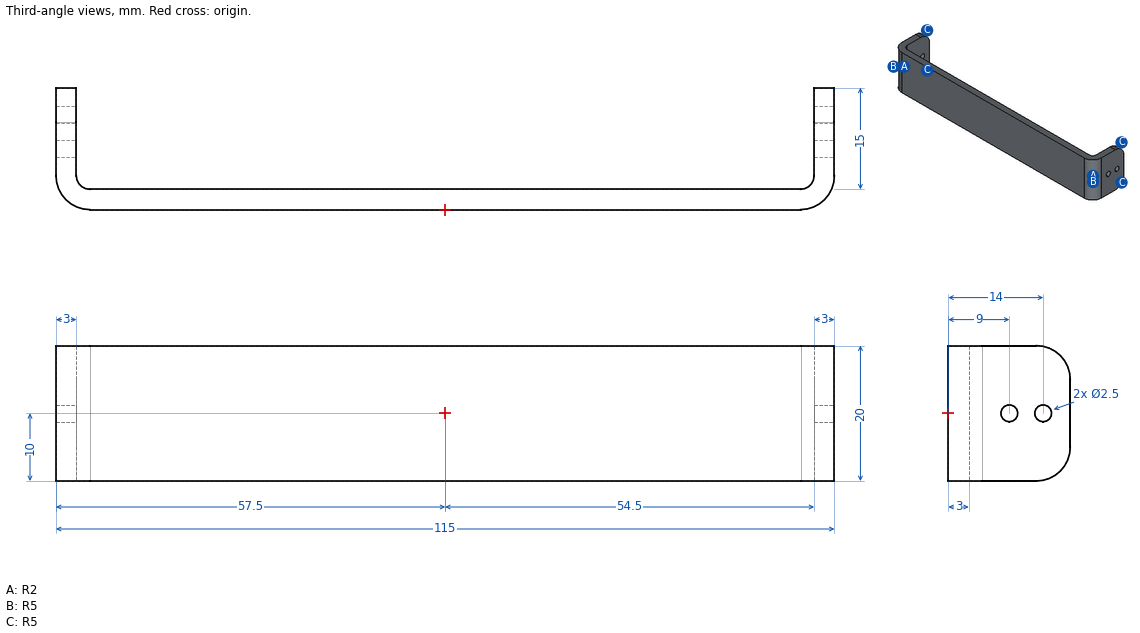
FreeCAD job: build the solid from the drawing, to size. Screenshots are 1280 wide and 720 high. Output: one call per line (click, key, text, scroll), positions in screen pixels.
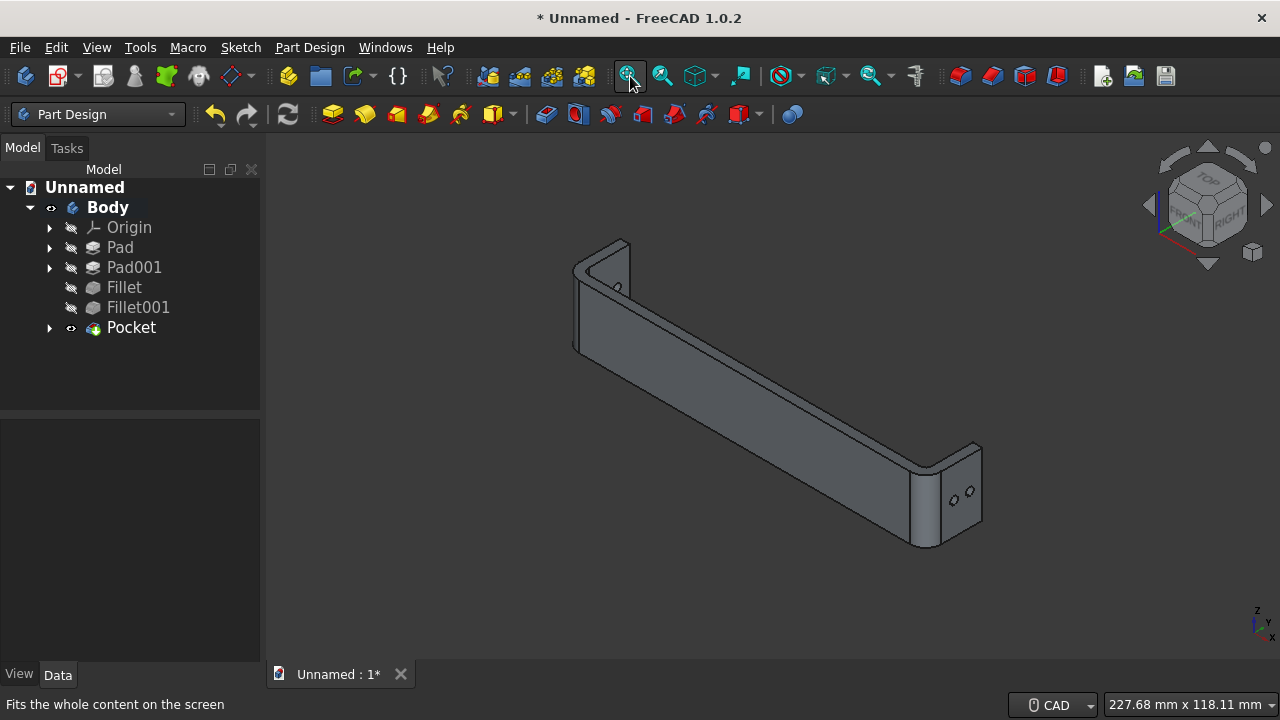
scroll(625, 240, up, 6)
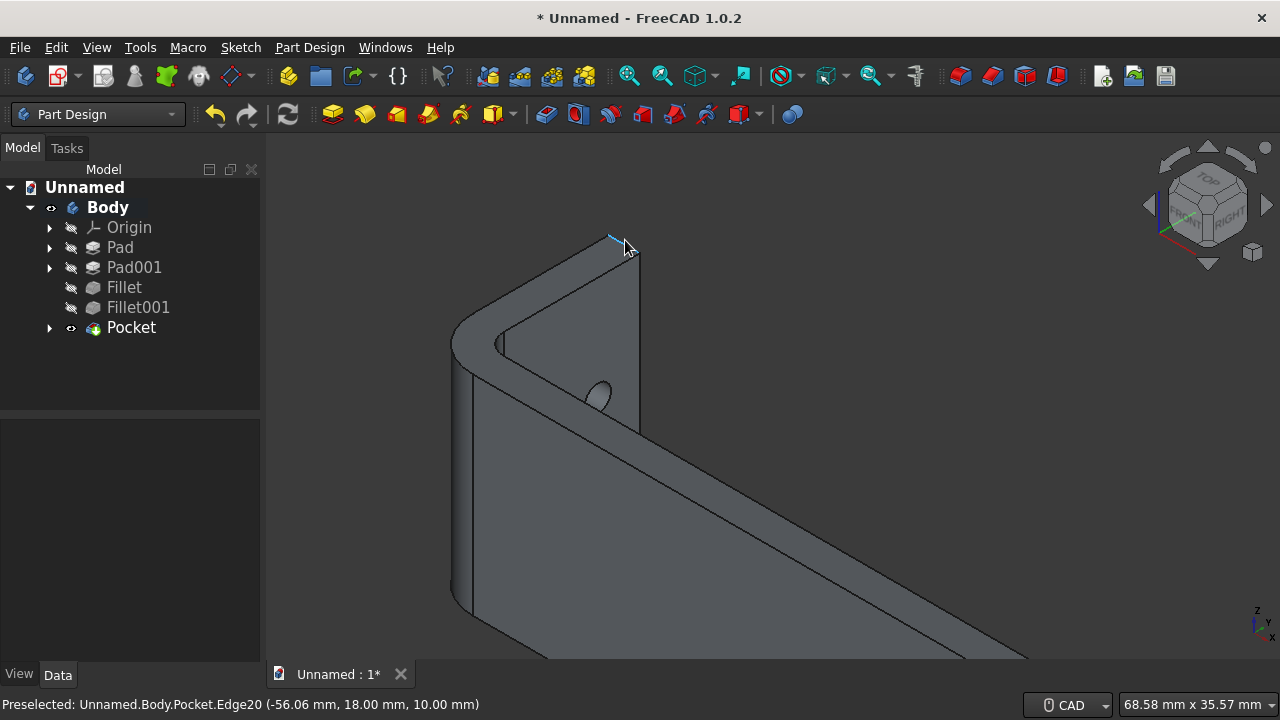
click(630, 76)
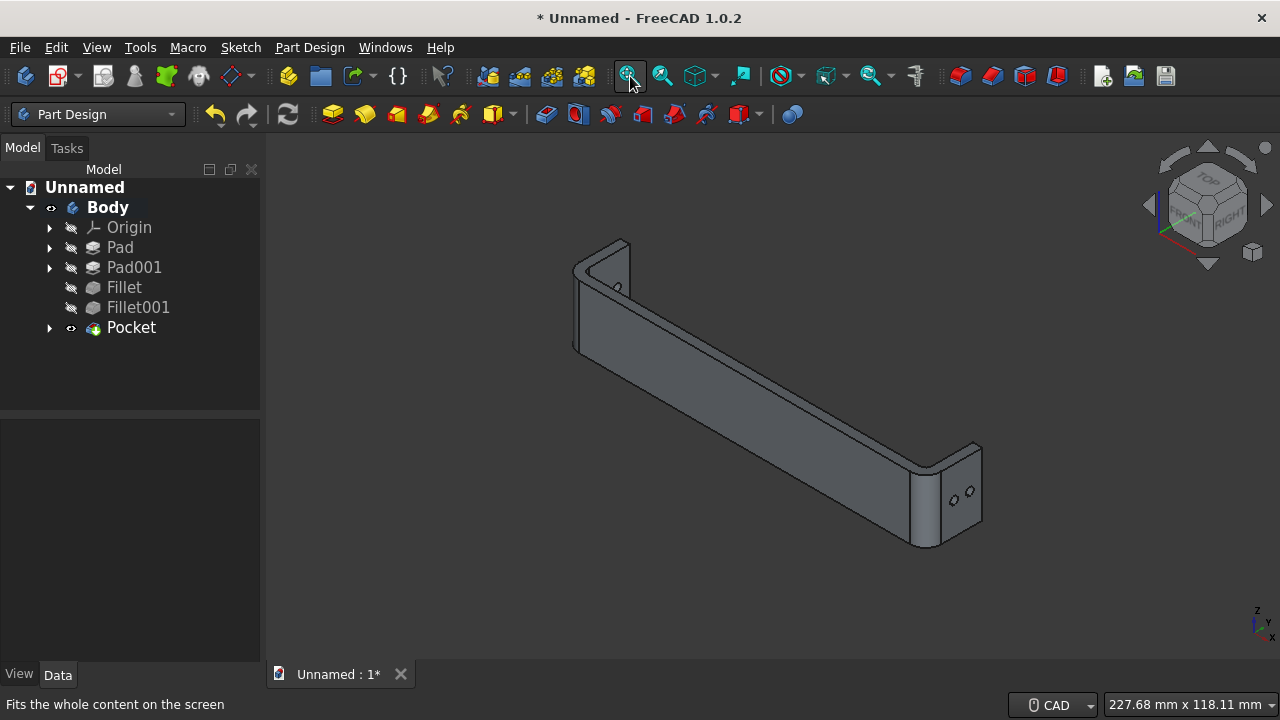
key(2)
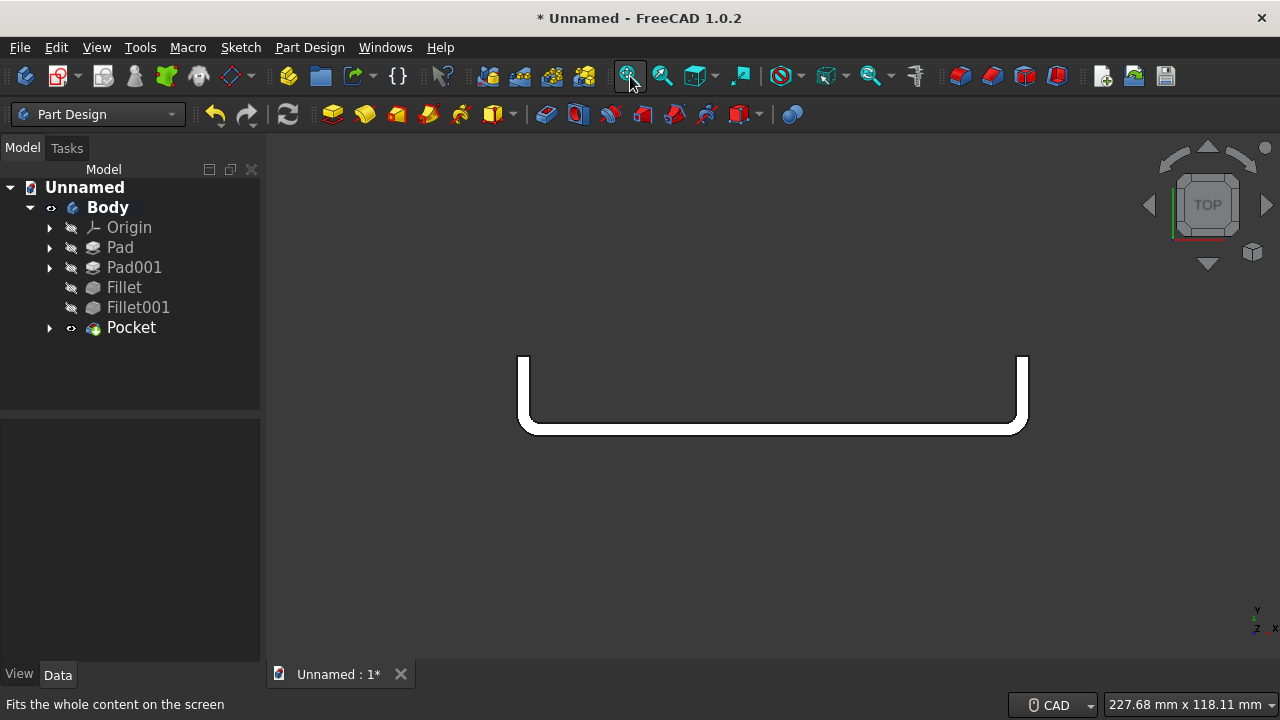
click(524, 355)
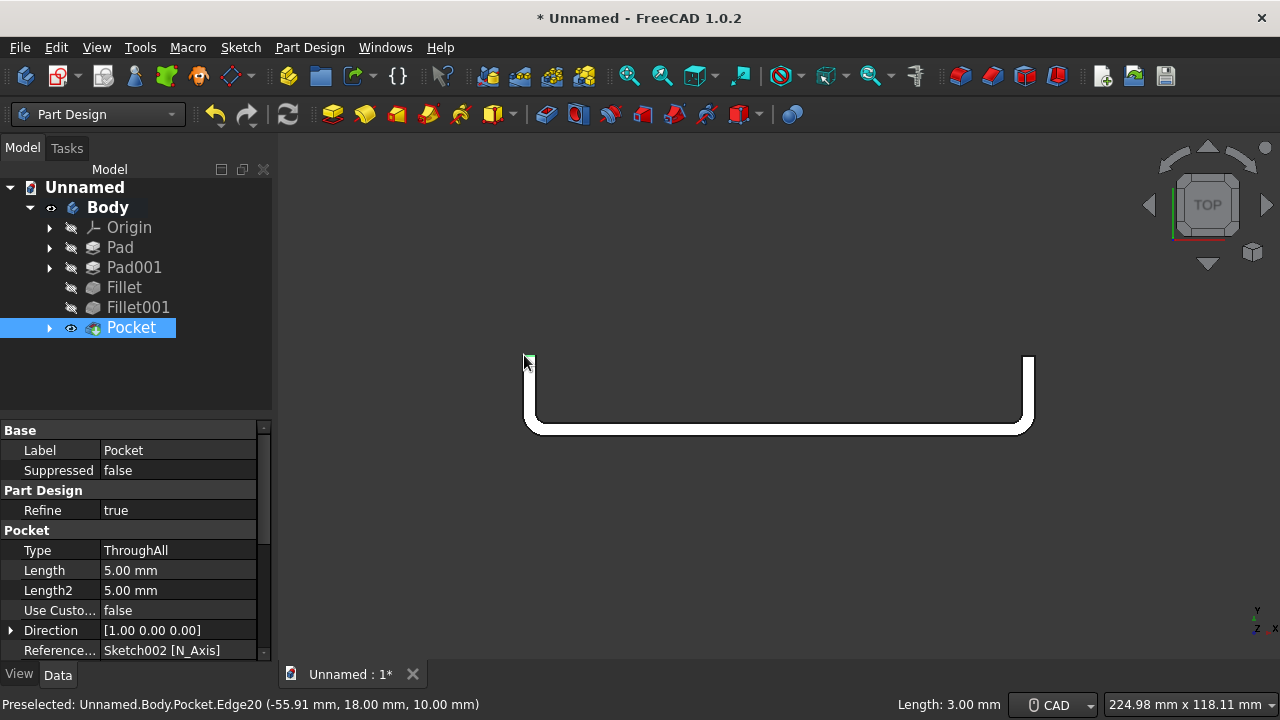
click(1028, 355, ctrl)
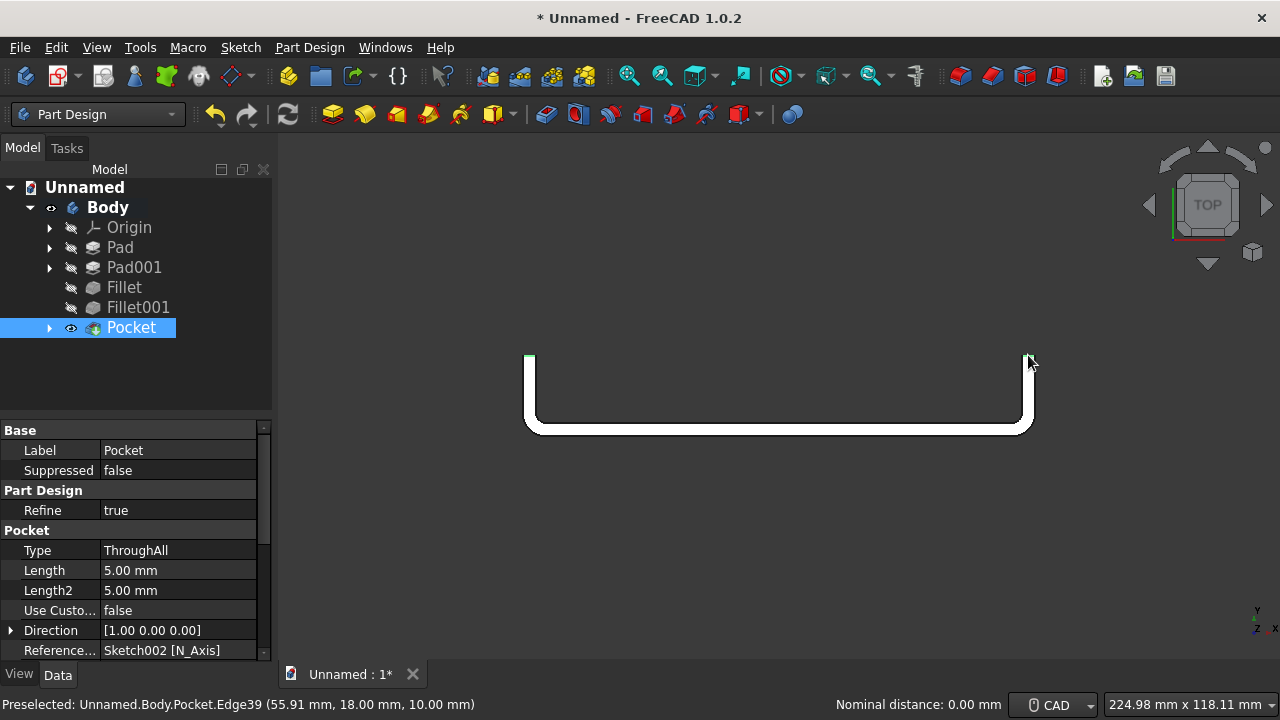
scroll(530, 355, up, 6)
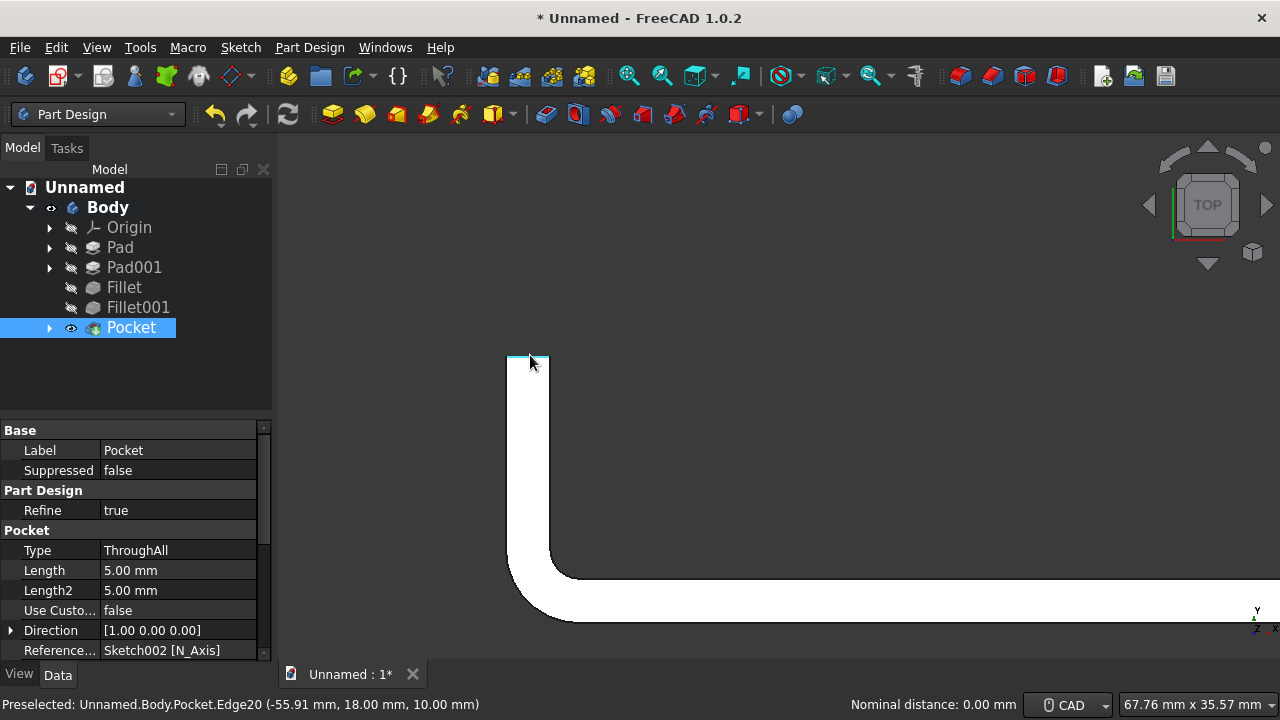
key(v)
key(f)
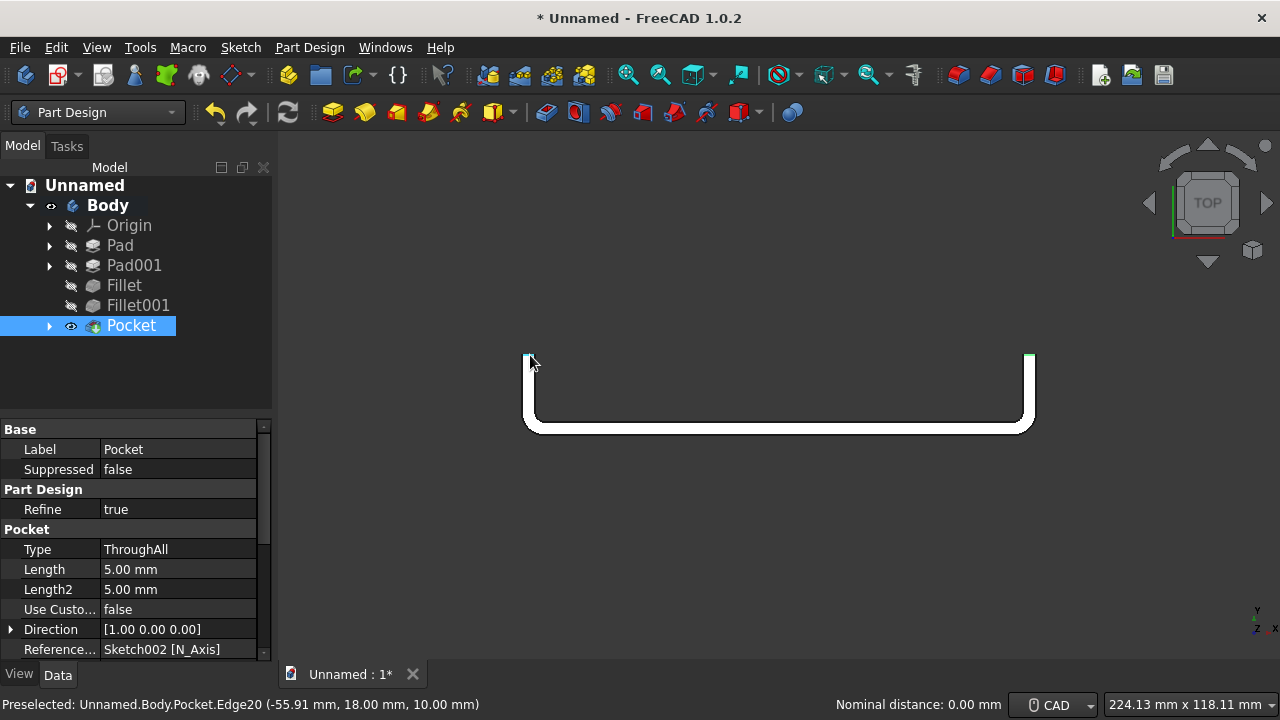
key(1)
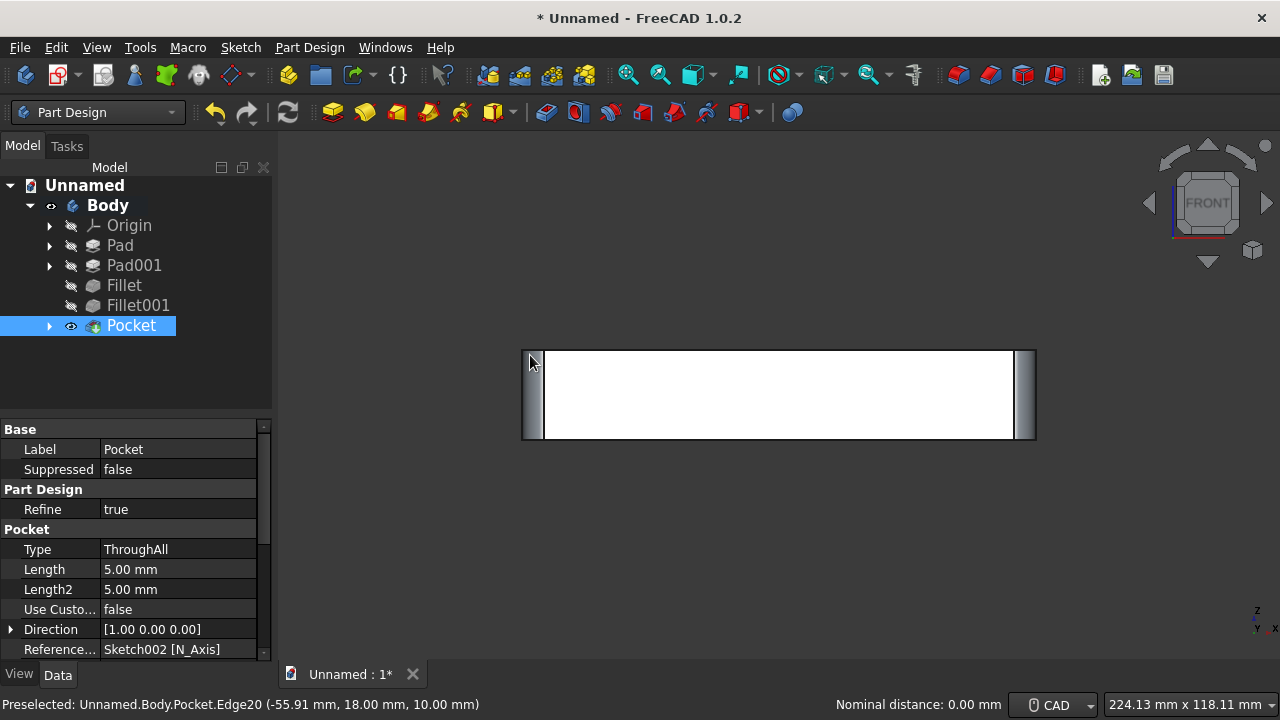
scroll(529, 439, up, 6)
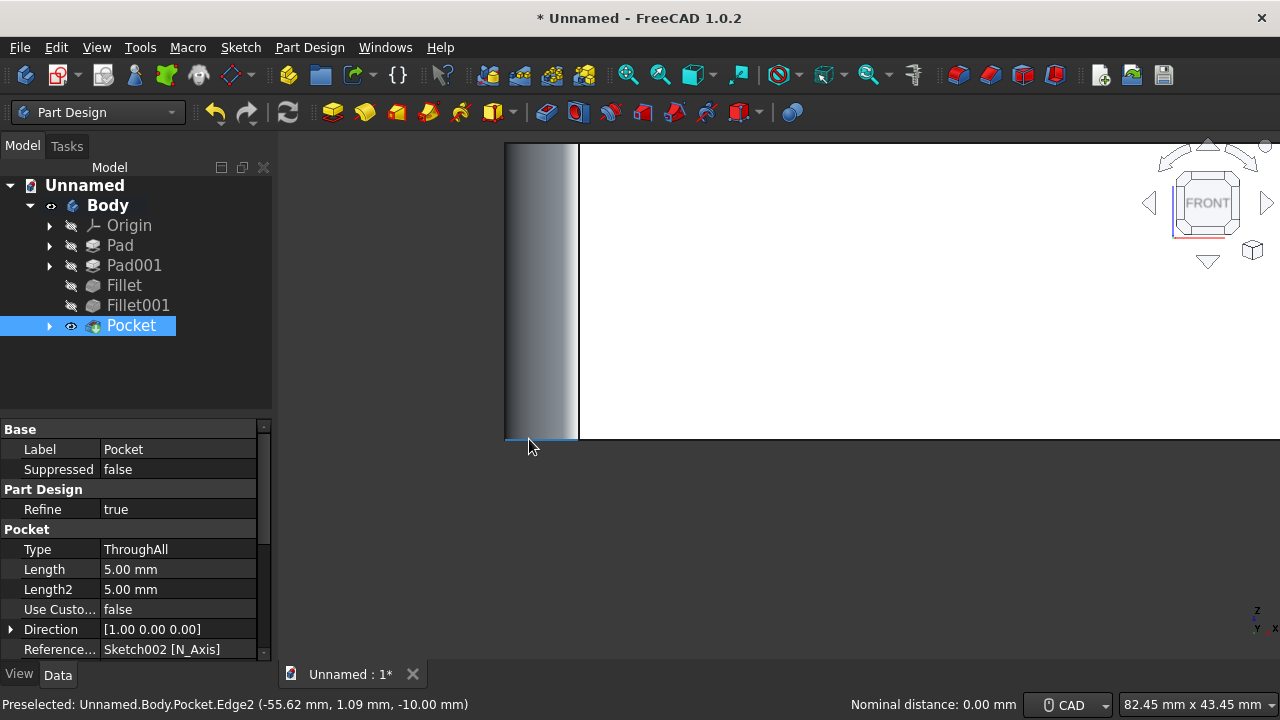
click(630, 76)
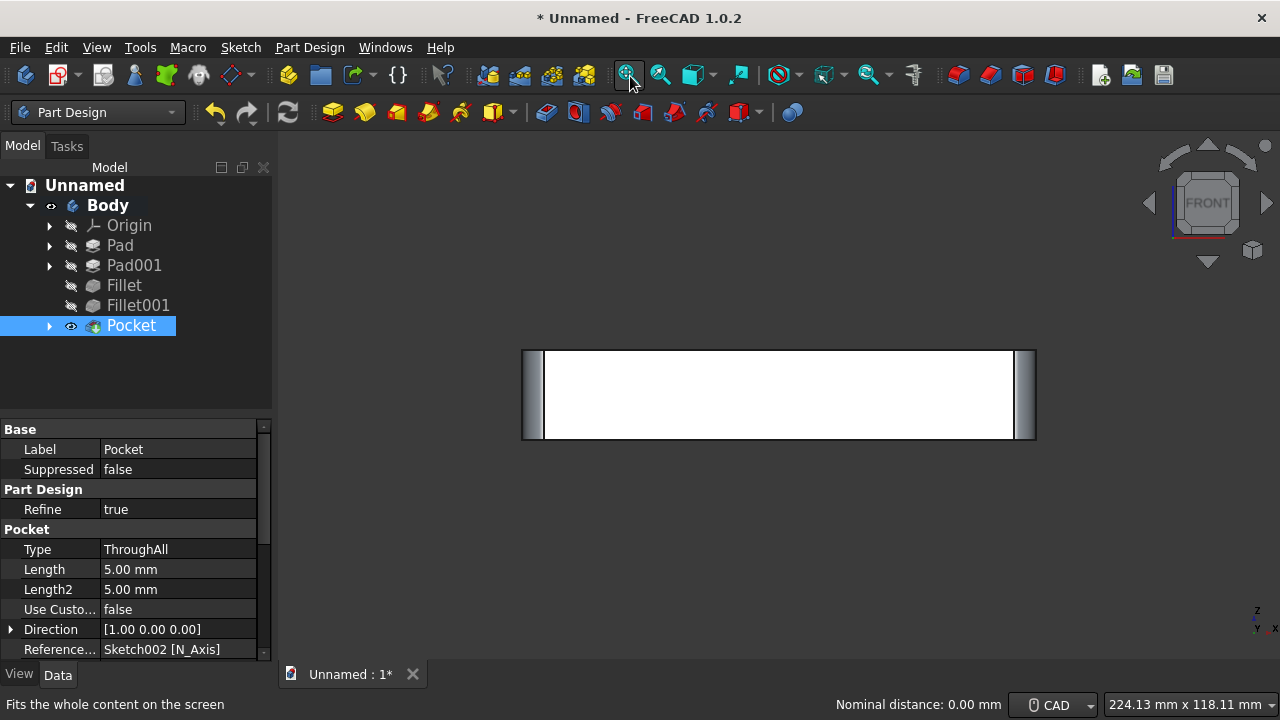
key(3)